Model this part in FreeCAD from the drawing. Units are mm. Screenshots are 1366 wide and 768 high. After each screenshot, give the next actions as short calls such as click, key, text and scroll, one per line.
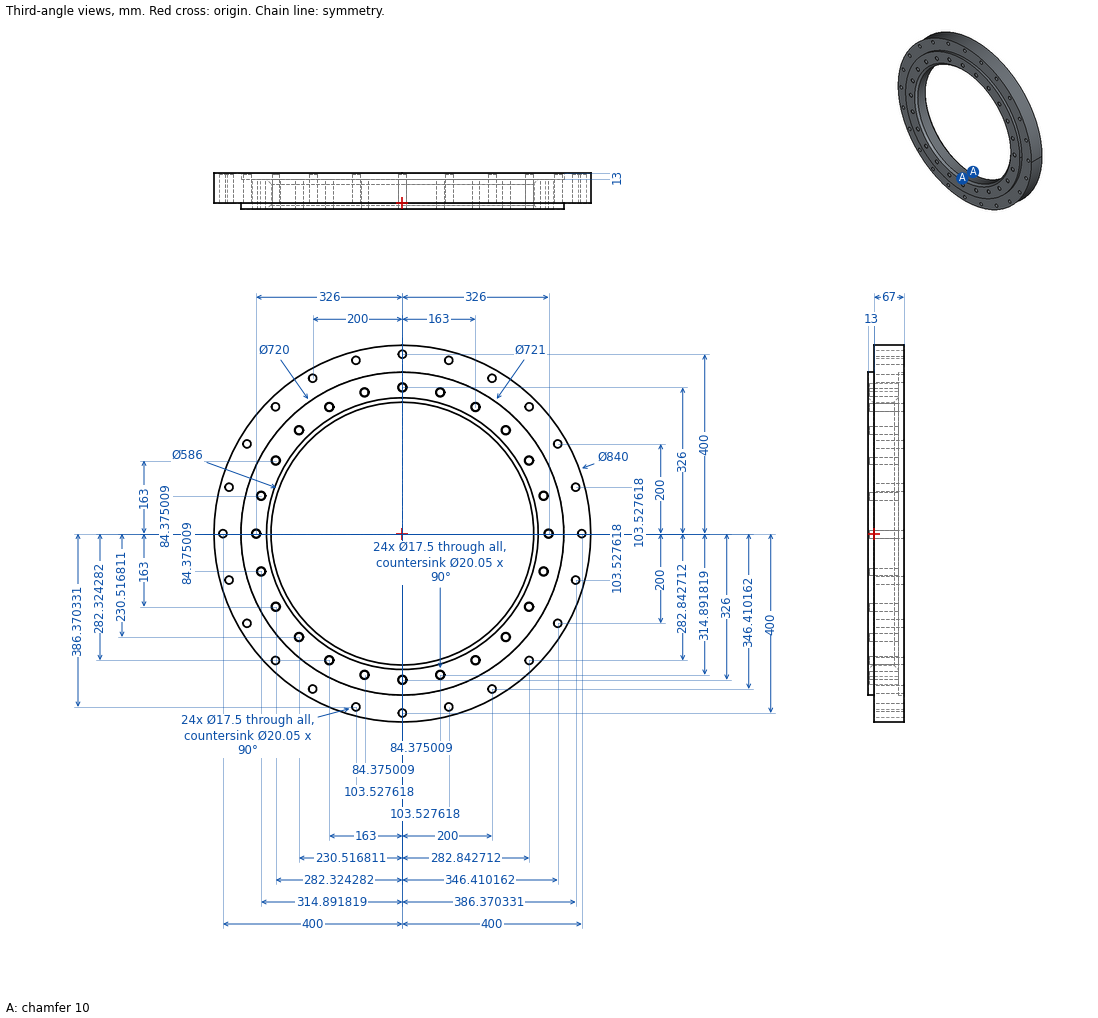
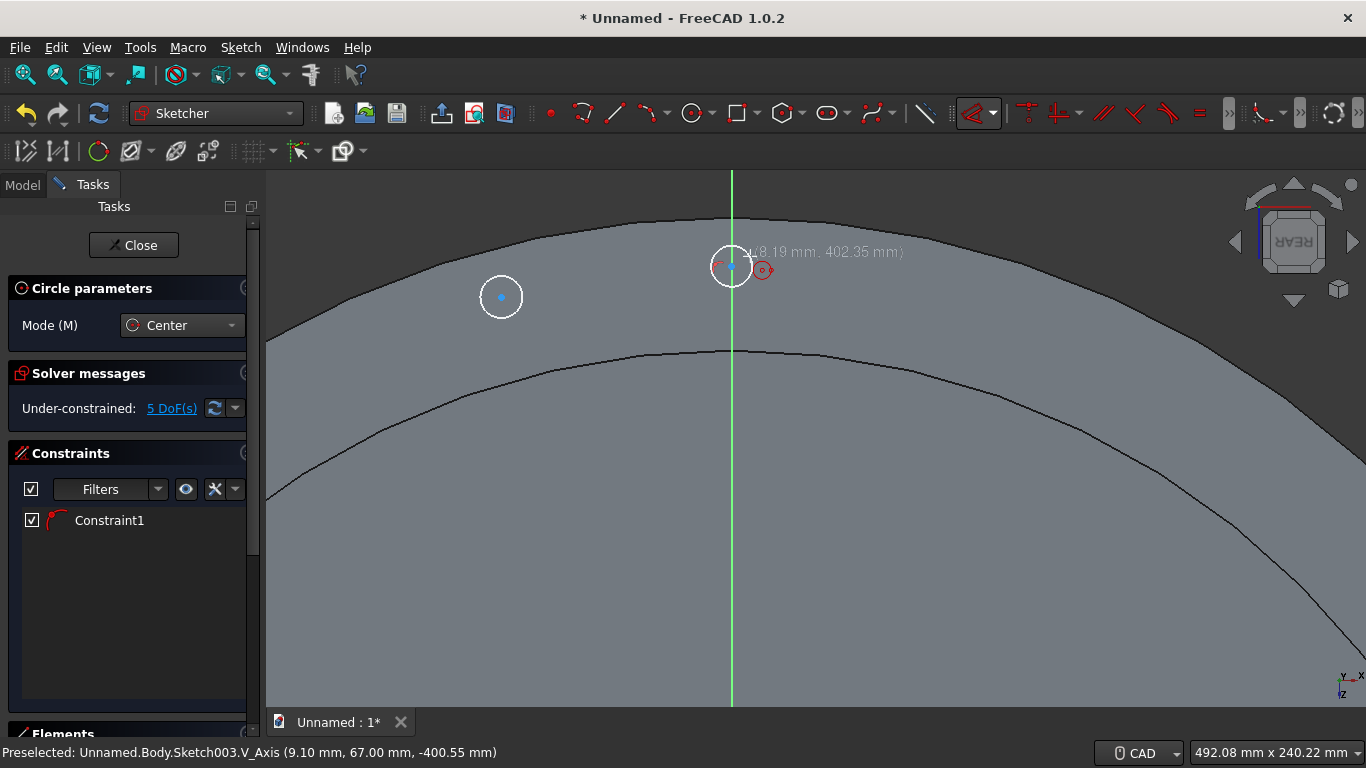
scroll(751, 257, down, 8)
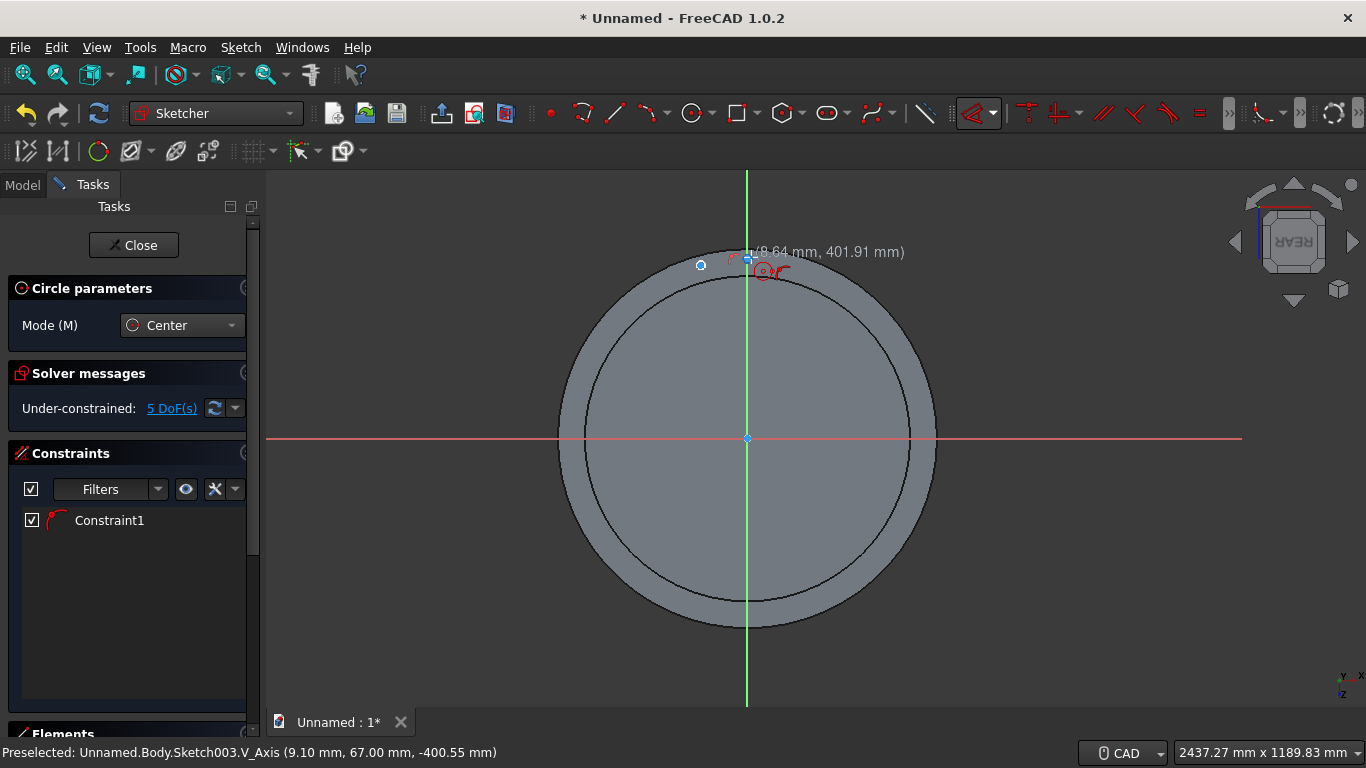
click(794, 264)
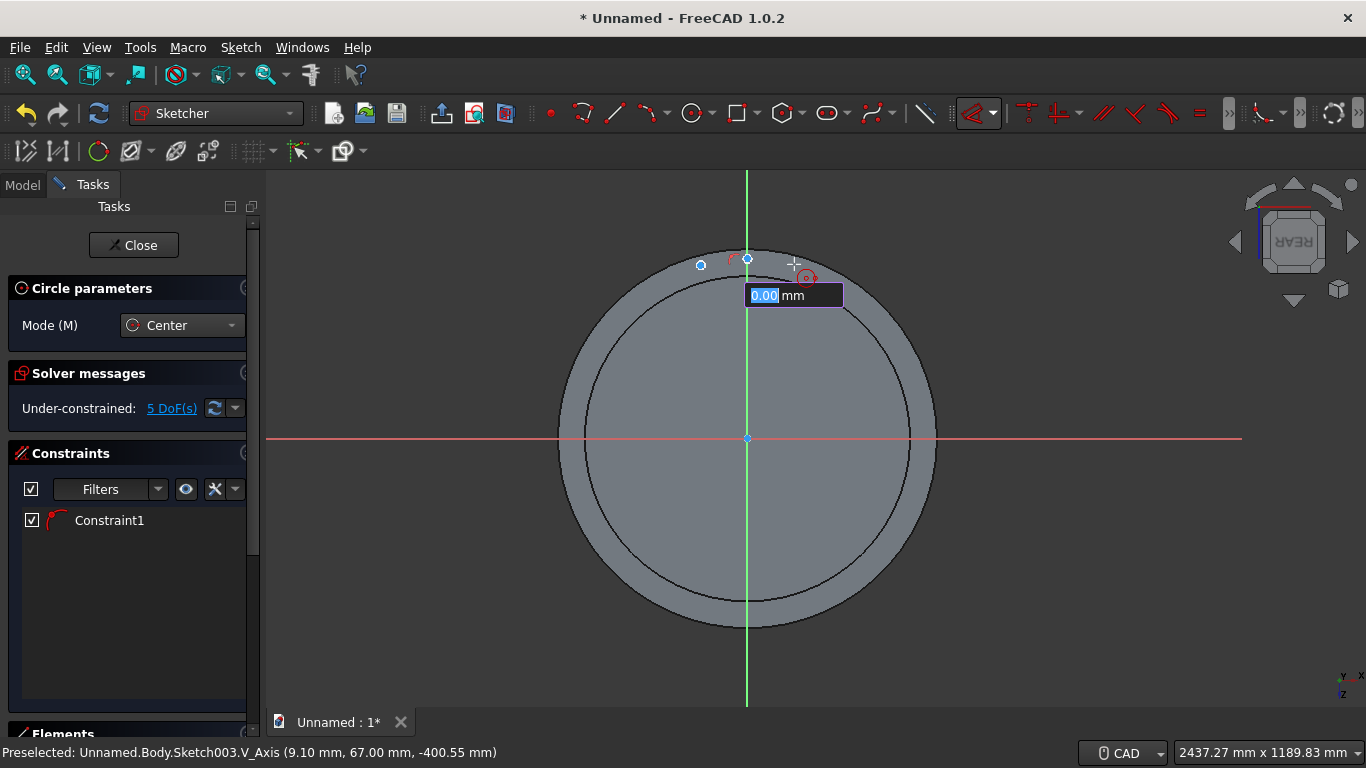
scroll(797, 262, up, 7)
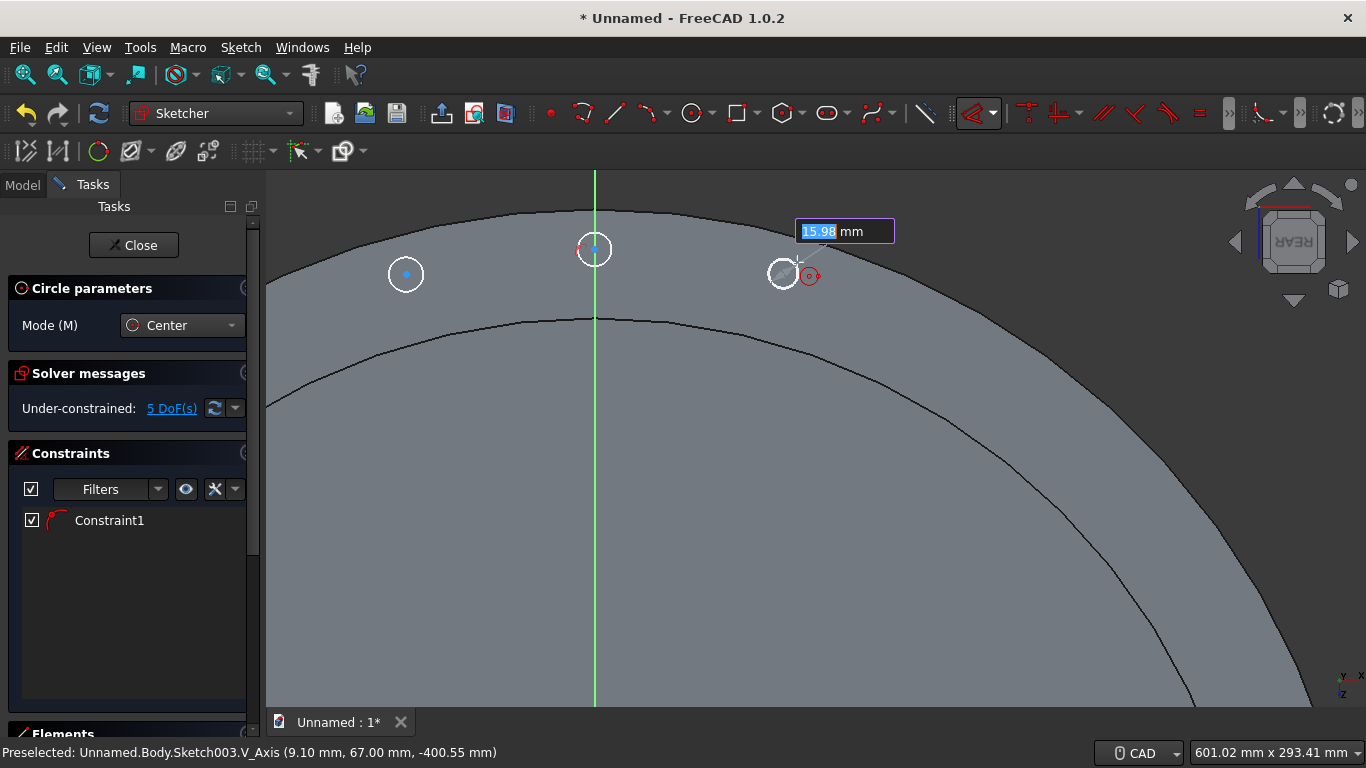
click(795, 260)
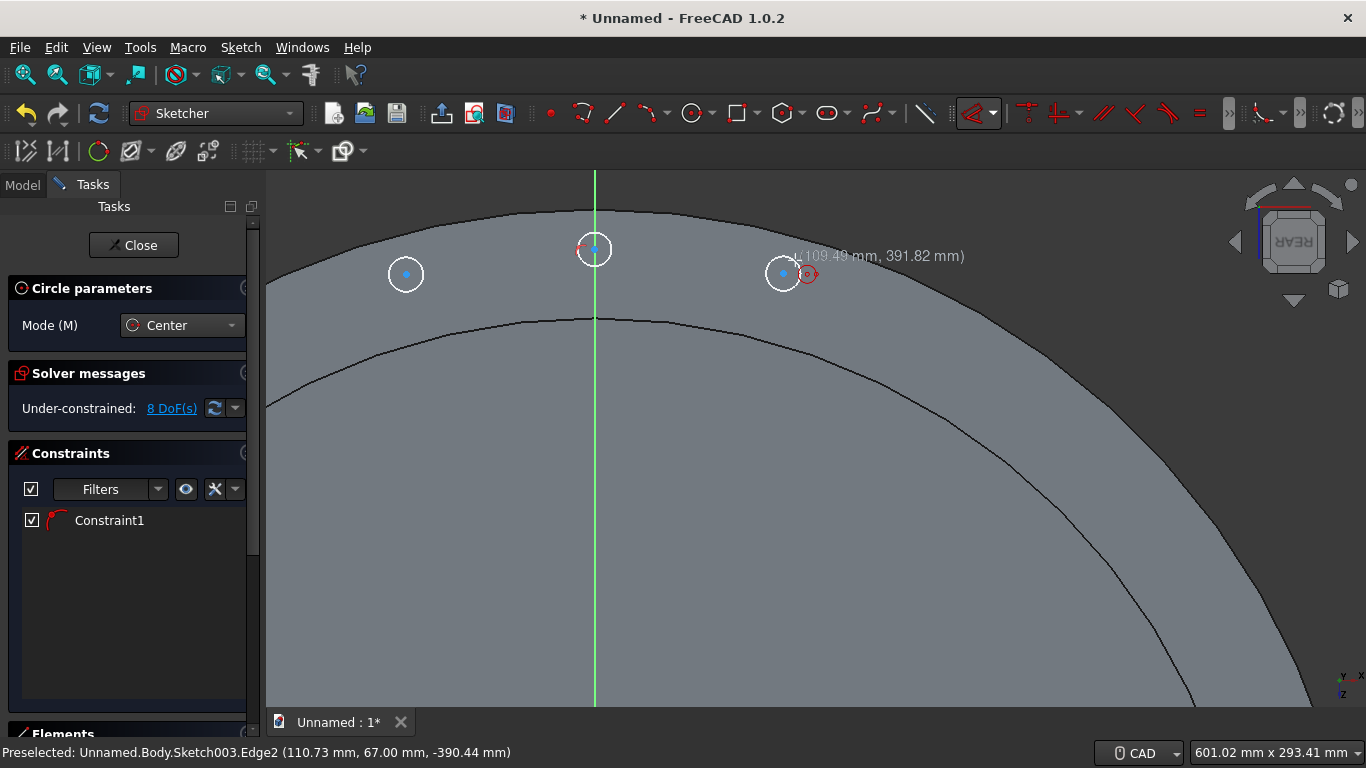
scroll(961, 344, up, 2)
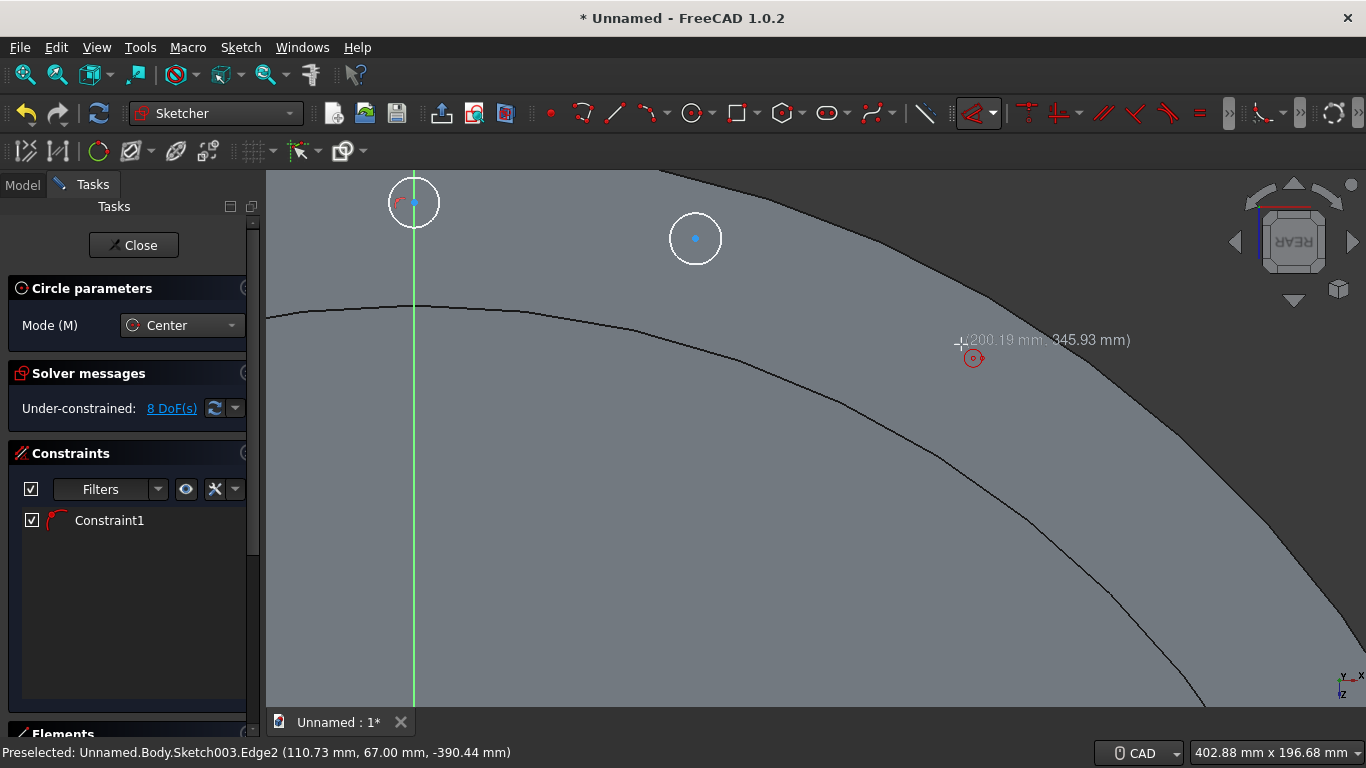
scroll(814, 270, down, 9)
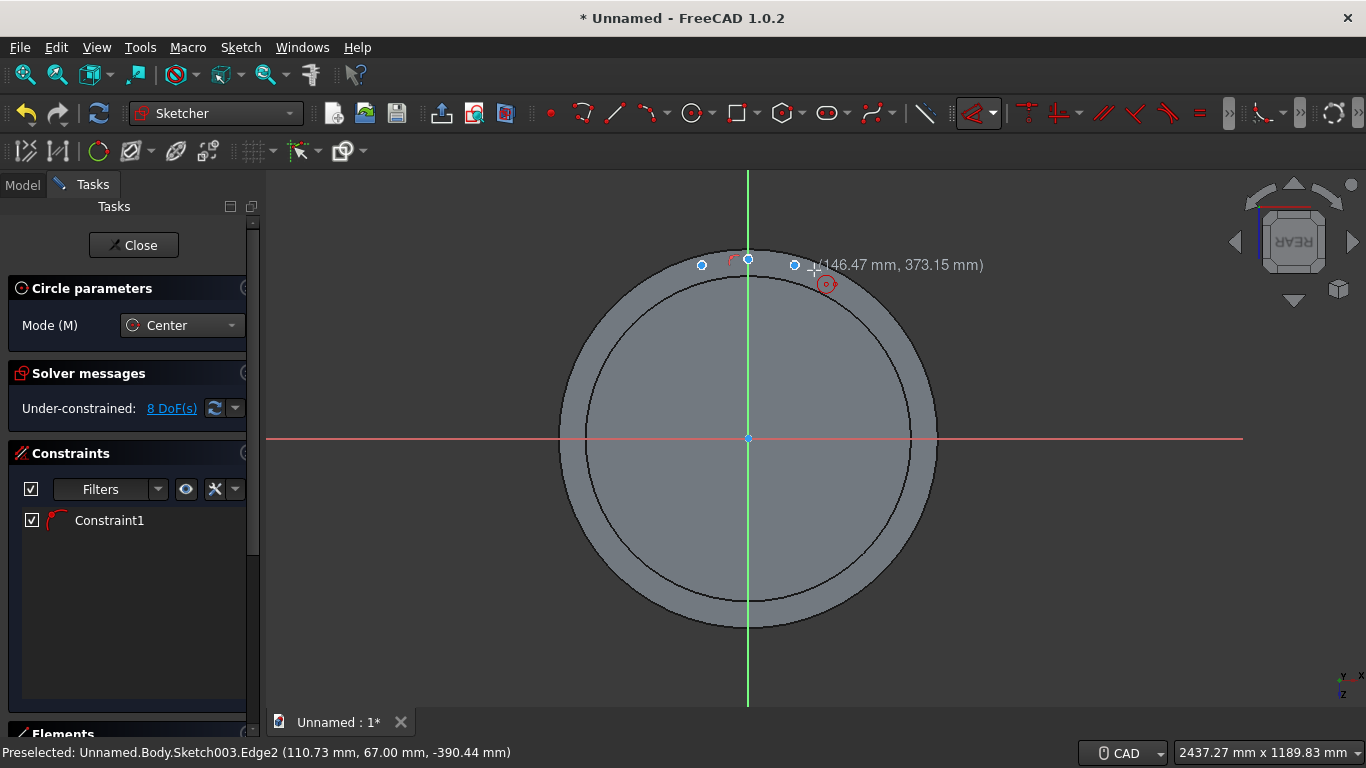
click(839, 282)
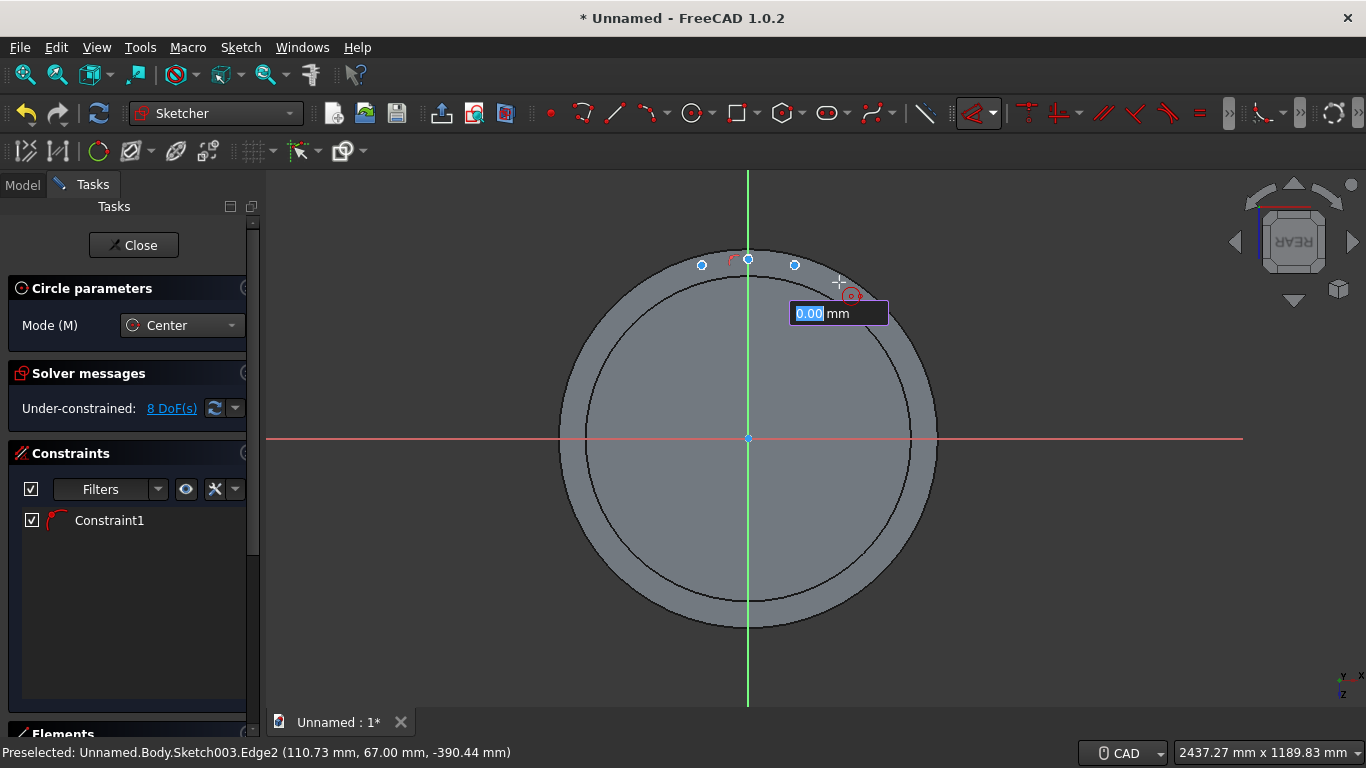
scroll(841, 280, up, 7)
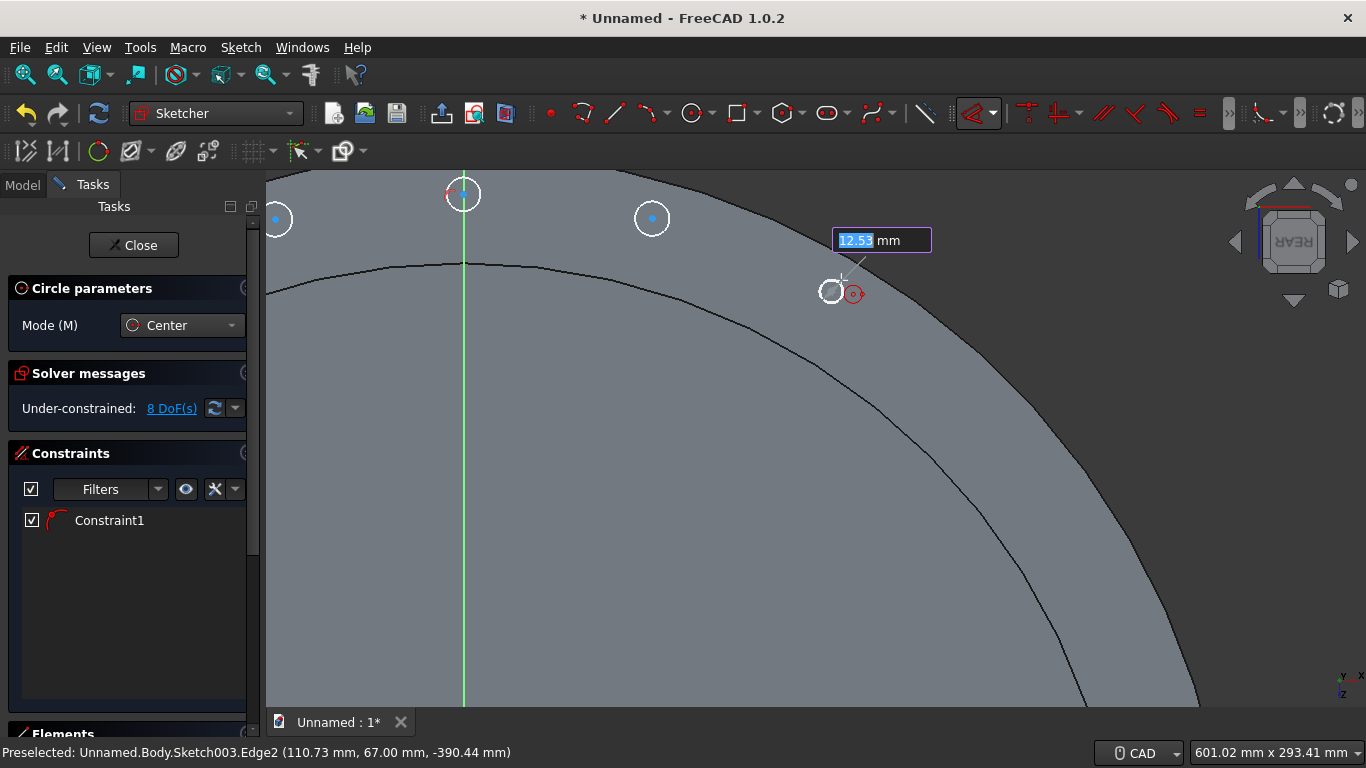
click(841, 278)